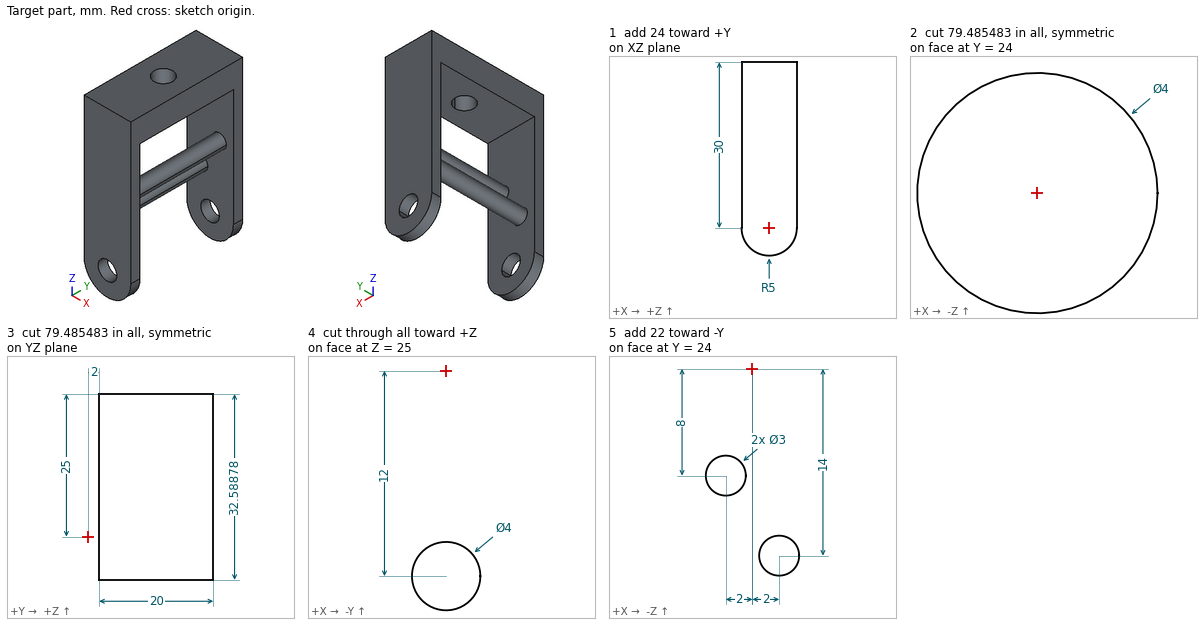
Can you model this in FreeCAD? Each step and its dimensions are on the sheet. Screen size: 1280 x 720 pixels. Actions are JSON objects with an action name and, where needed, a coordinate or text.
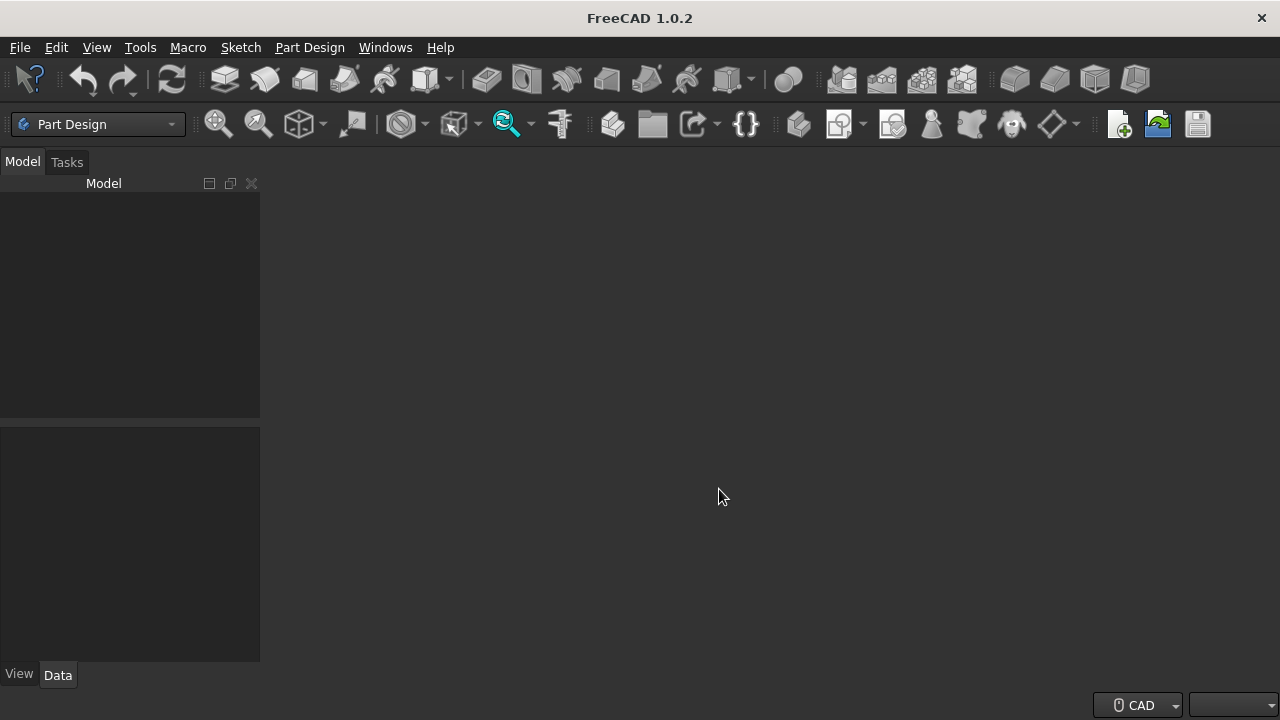
{"action": "left_click", "coordinate": [1118, 124]}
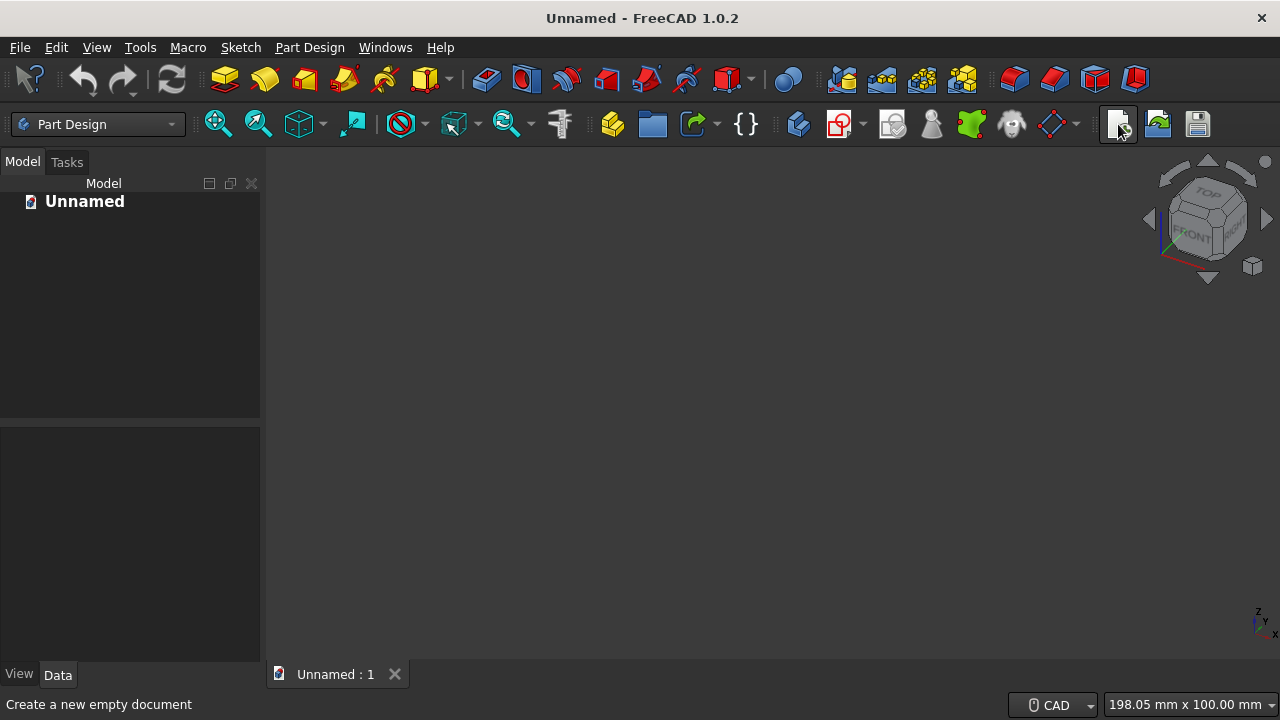
{"action": "left_click", "coordinate": [840, 124]}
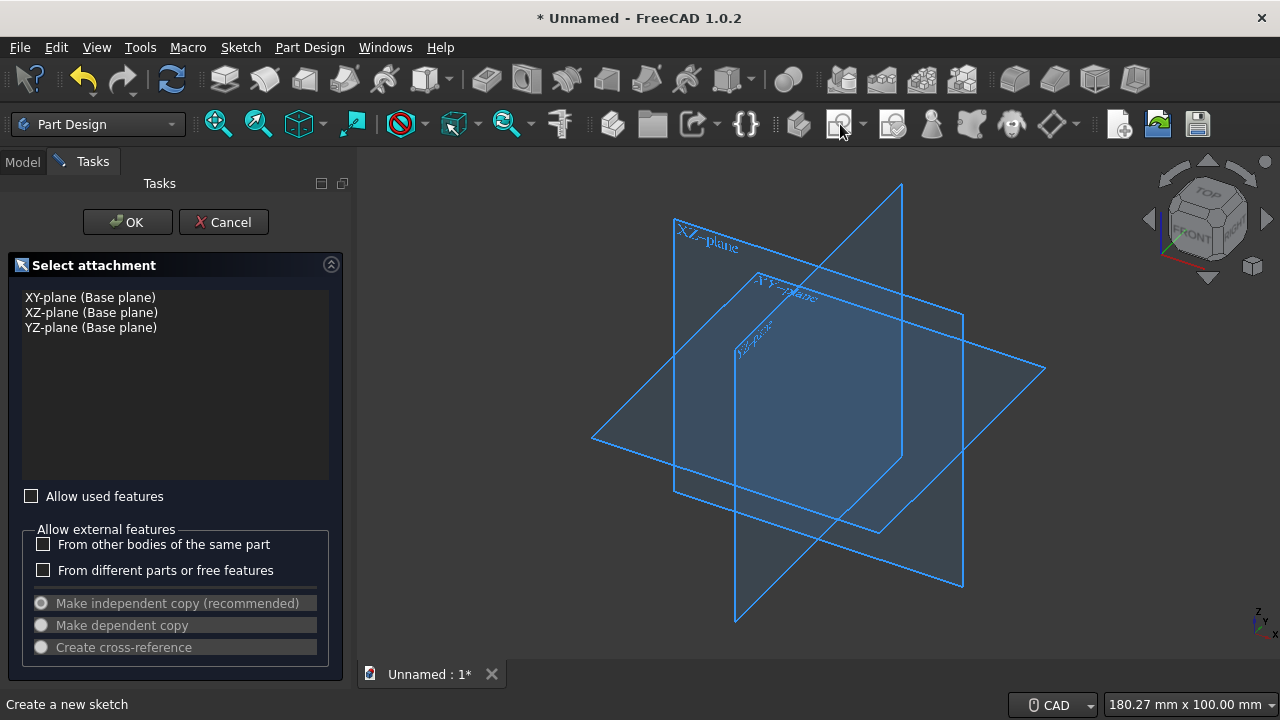
{"action": "left_click", "coordinate": [82, 312]}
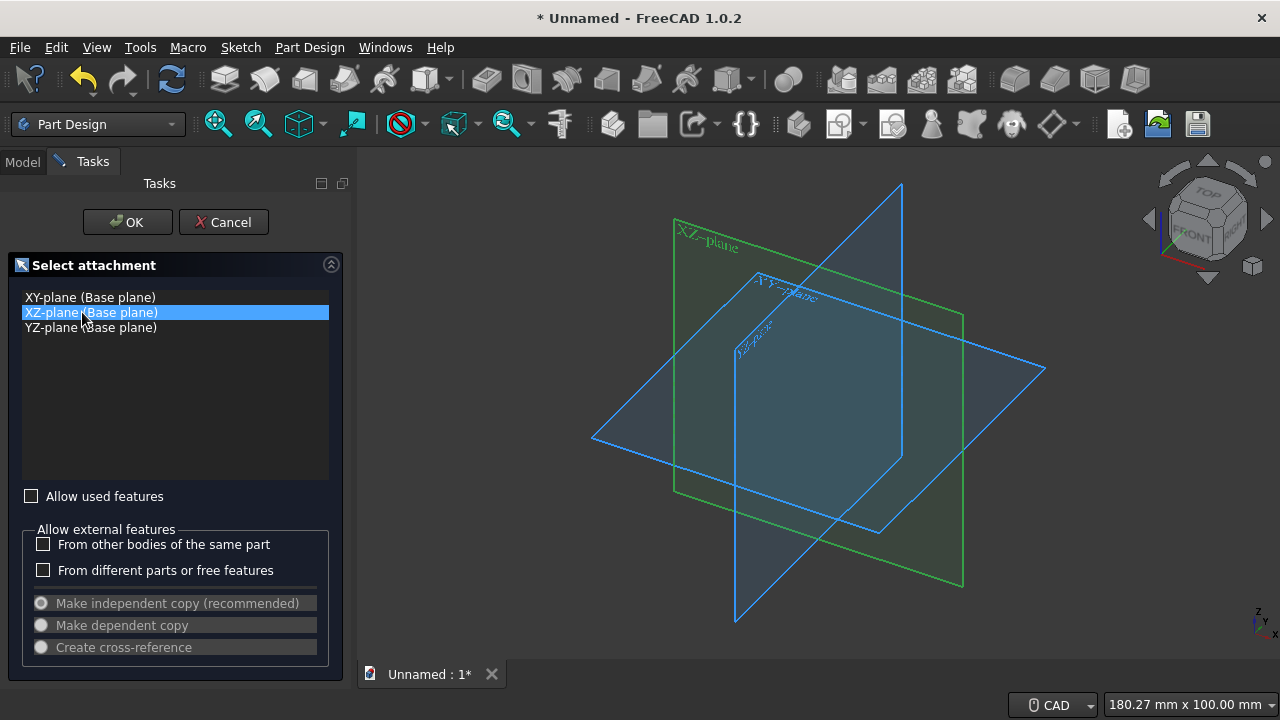
{"action": "left_click", "coordinate": [128, 222]}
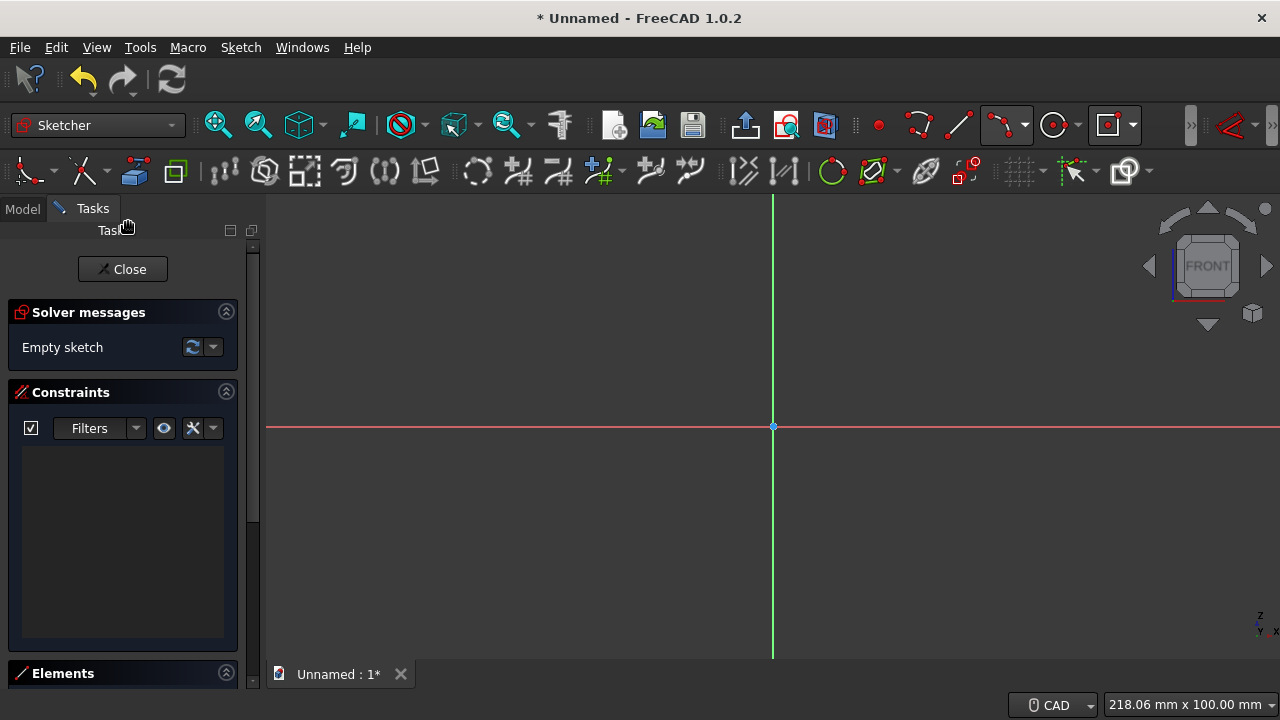
{"action": "scroll", "coordinate": [856, 298], "scroll_direction": "up", "scroll_amount": 3}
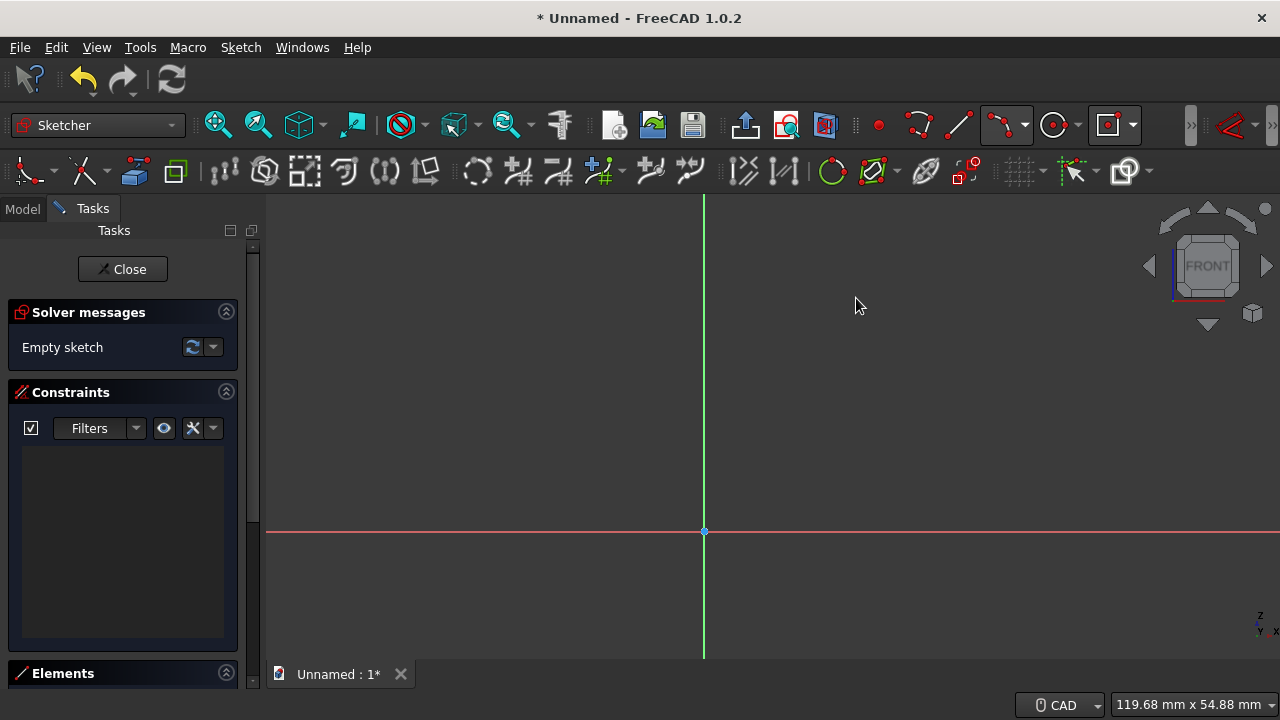
{"action": "left_click", "coordinate": [920, 126]}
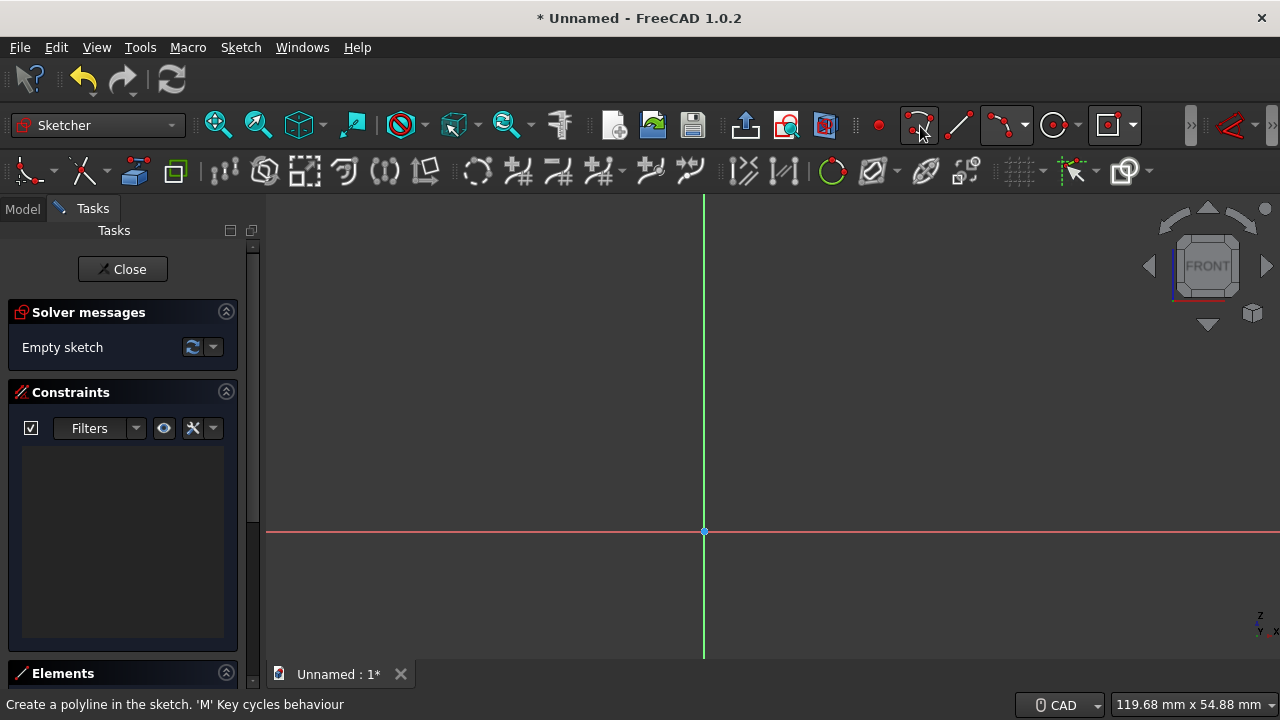
{"action": "left_click", "coordinate": [662, 532]}
{"action": "left_click", "coordinate": [662, 278]}
{"action": "left_click", "coordinate": [747, 278]}
{"action": "left_click", "coordinate": [747, 532]}
{"action": "right_click", "coordinate": [747, 532]}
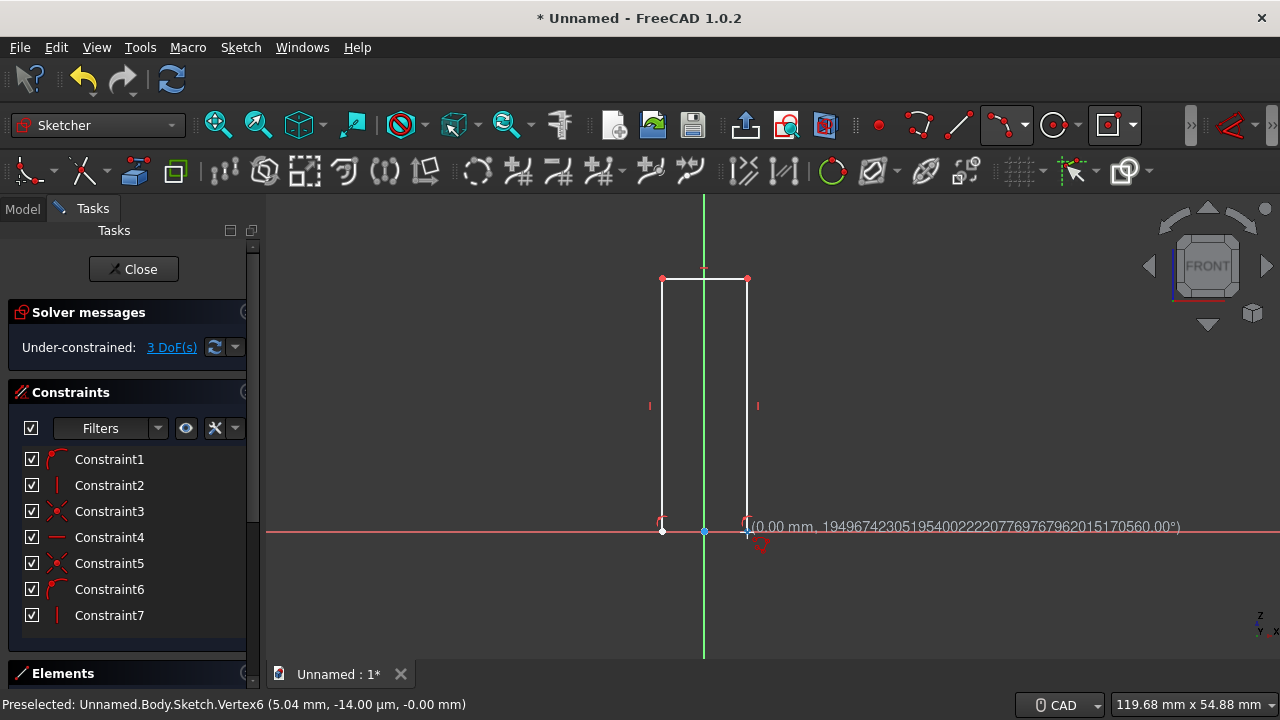
{"action": "left_click", "coordinate": [1000, 126]}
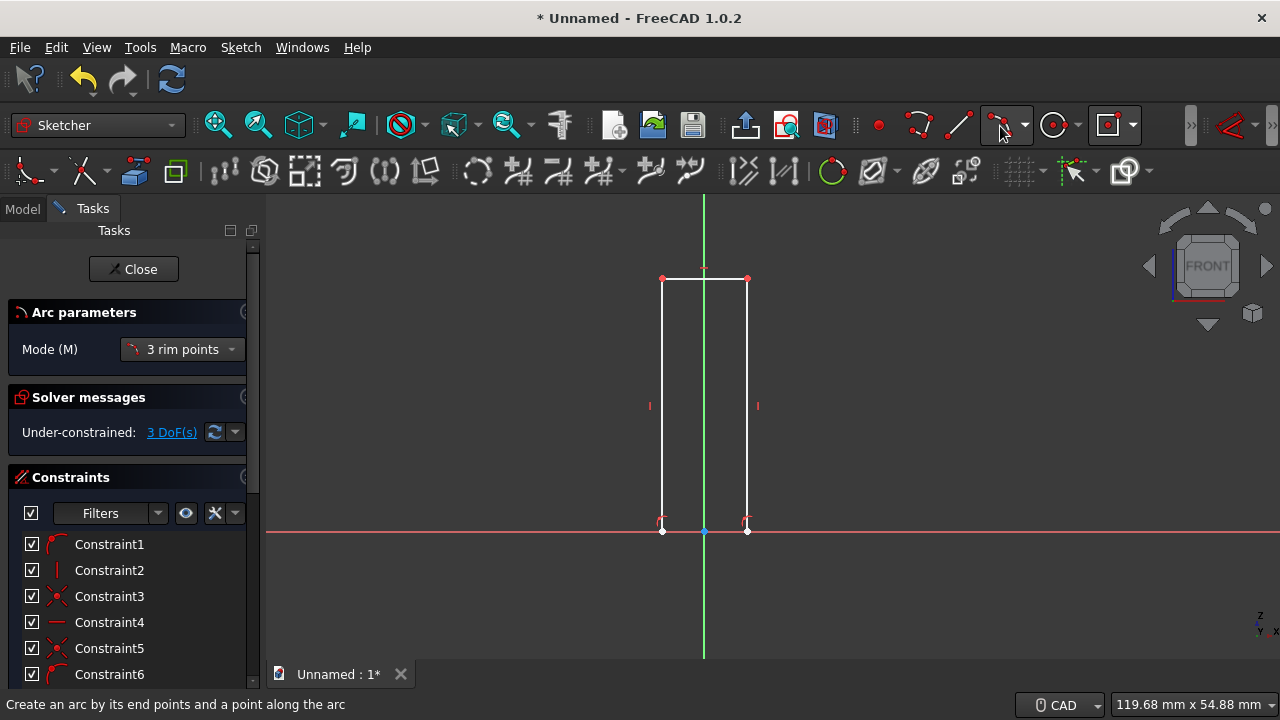
{"action": "left_click", "coordinate": [747, 532]}
{"action": "left_click", "coordinate": [662, 532]}
{"action": "left_click", "coordinate": [679, 566]}
{"action": "key", "text": "Escape"}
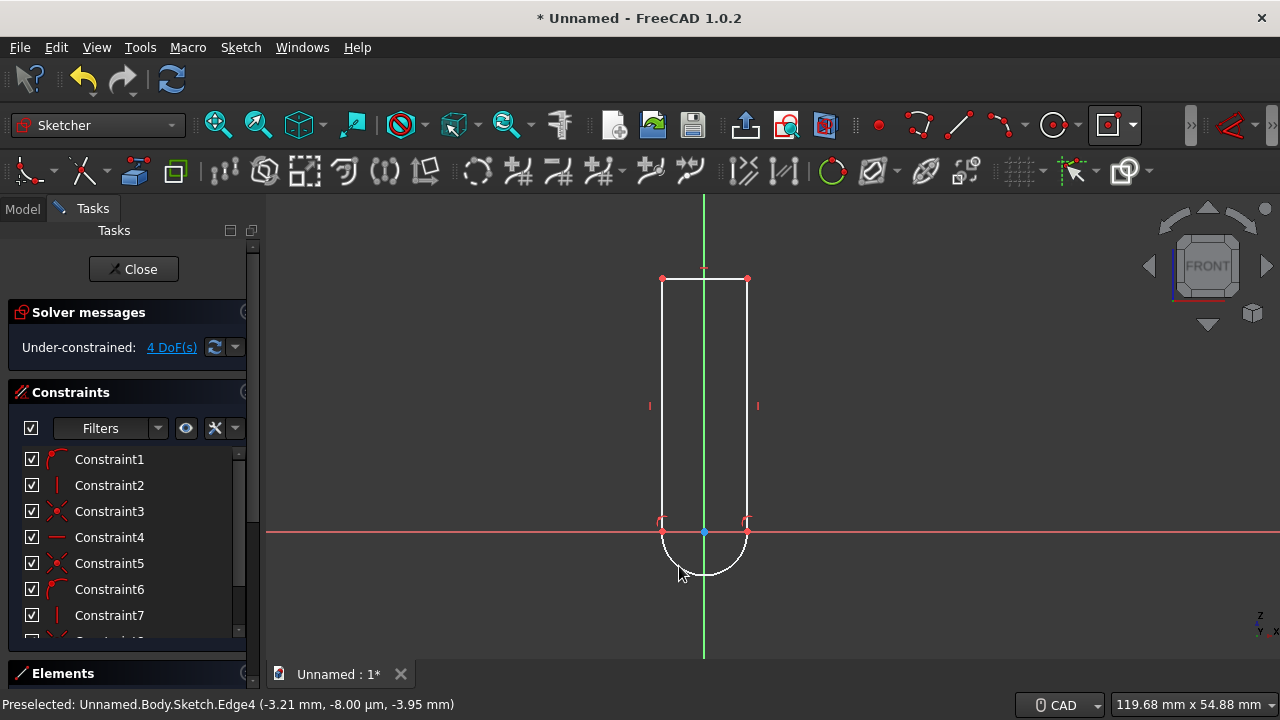
{"action": "left_click", "coordinate": [662, 456]}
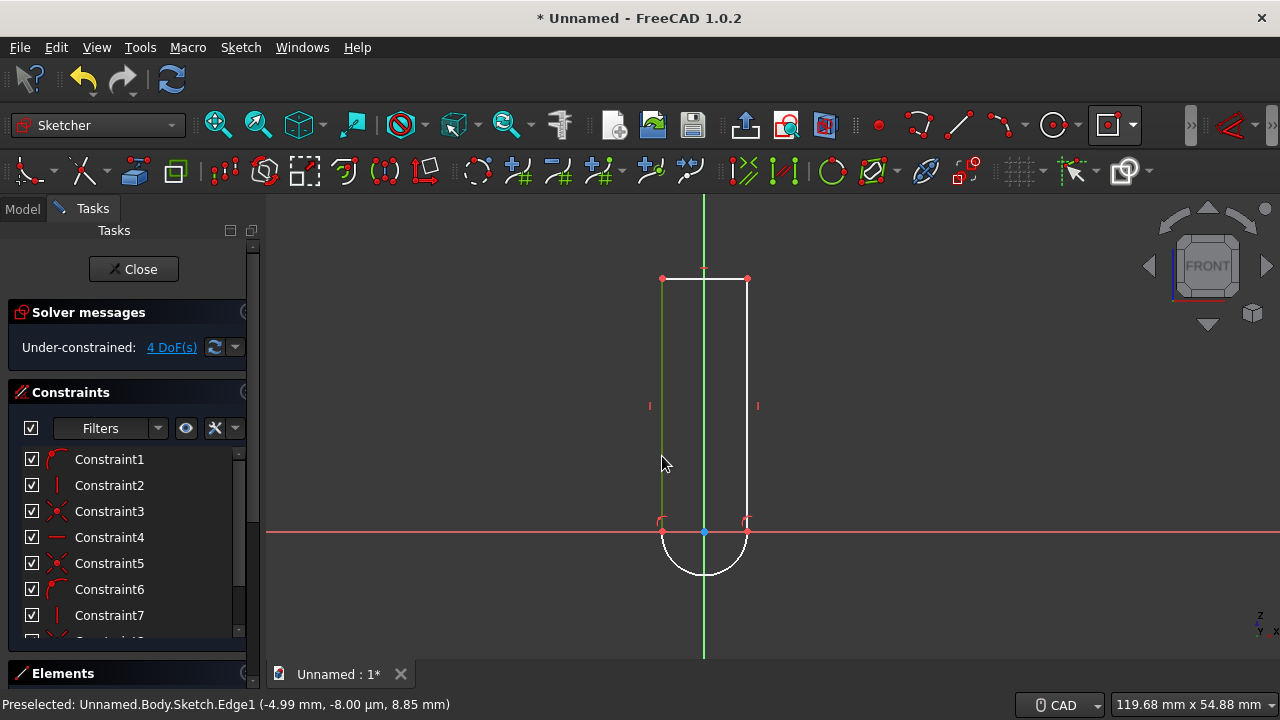
{"action": "left_click", "coordinate": [679, 567]}